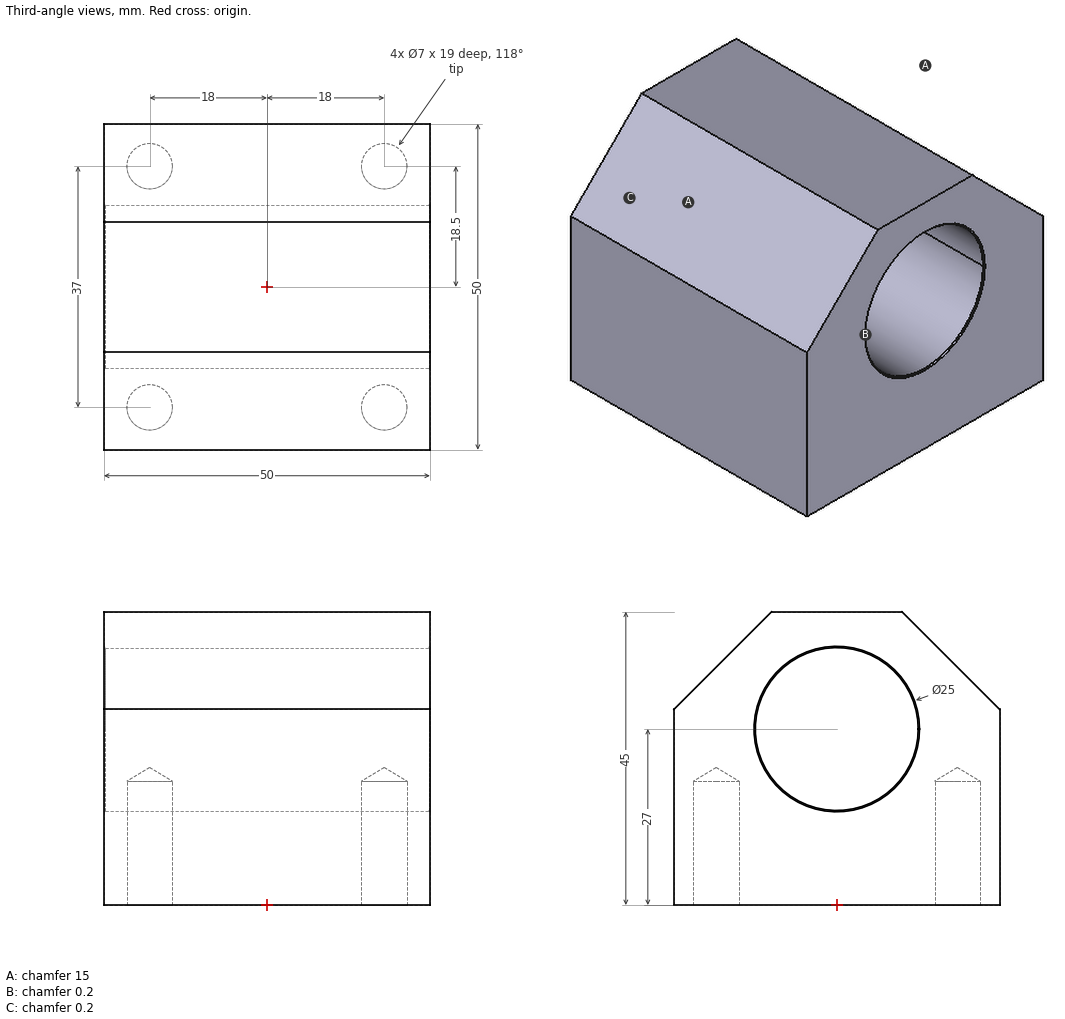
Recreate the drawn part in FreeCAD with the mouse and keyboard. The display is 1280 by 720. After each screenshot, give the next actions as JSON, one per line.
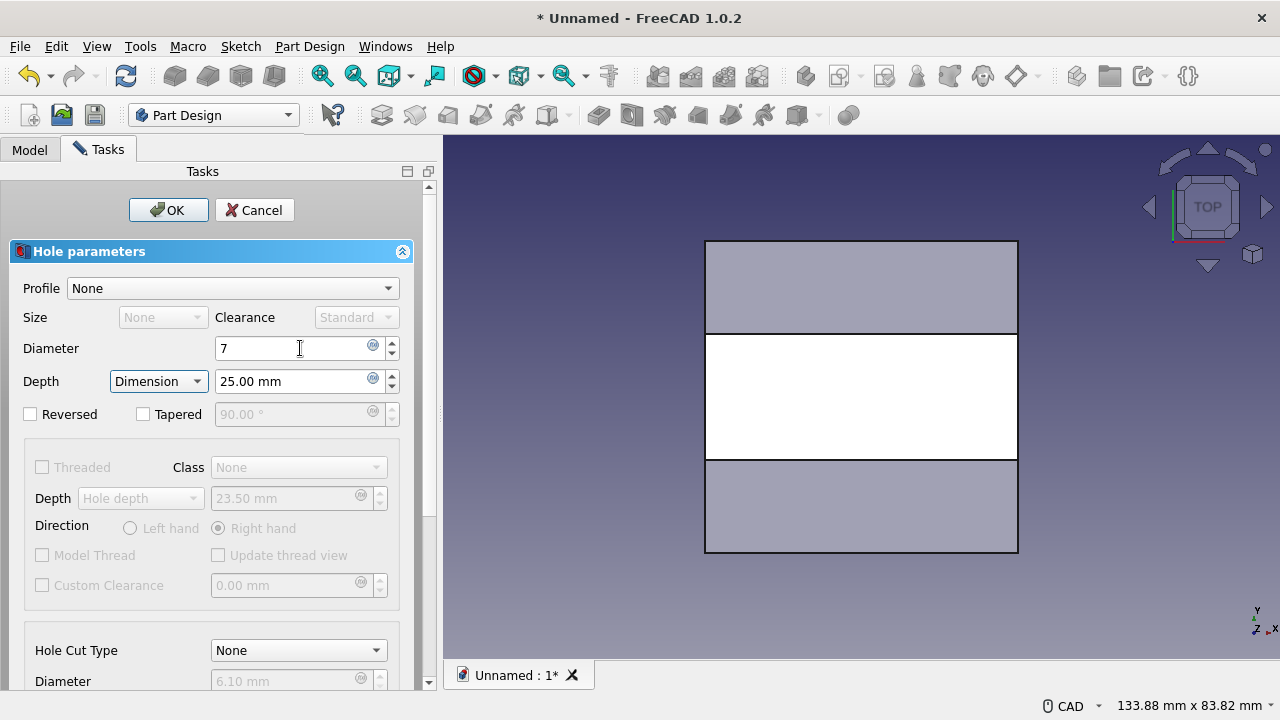
{"action": "triple_click", "coordinate": [300, 382]}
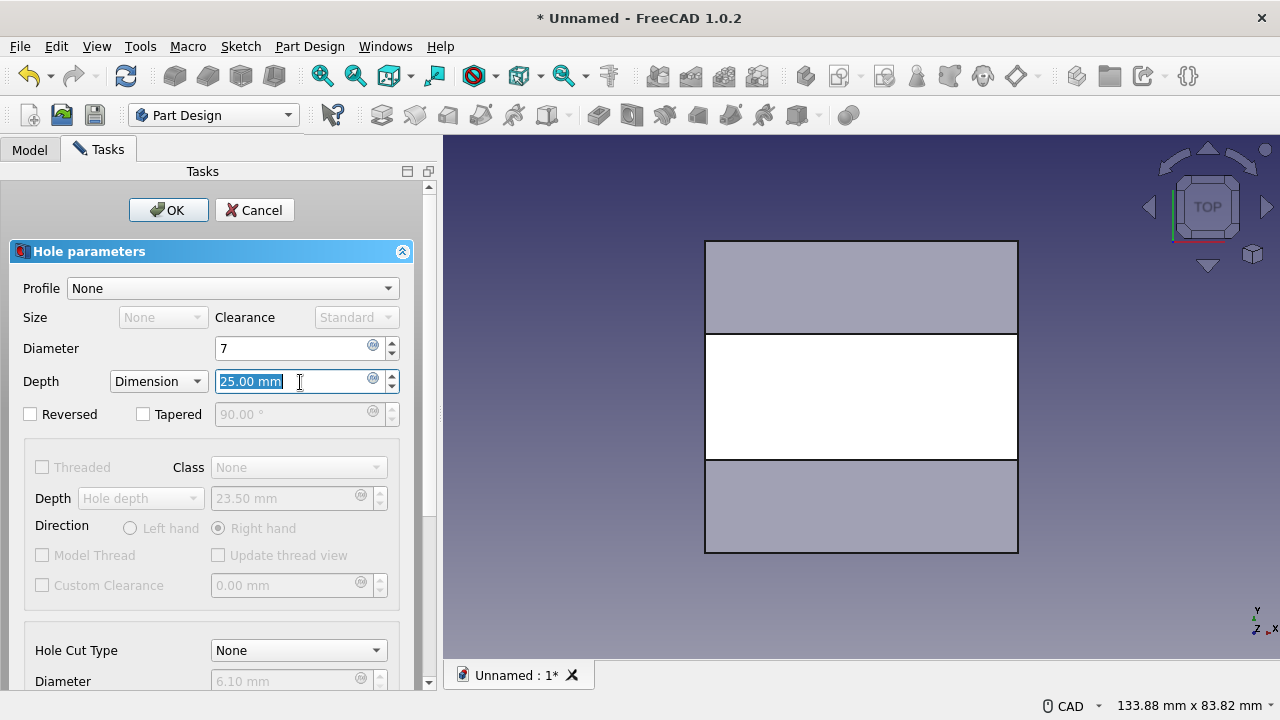
{"action": "type", "text": "19"}
{"action": "key", "text": "Tab"}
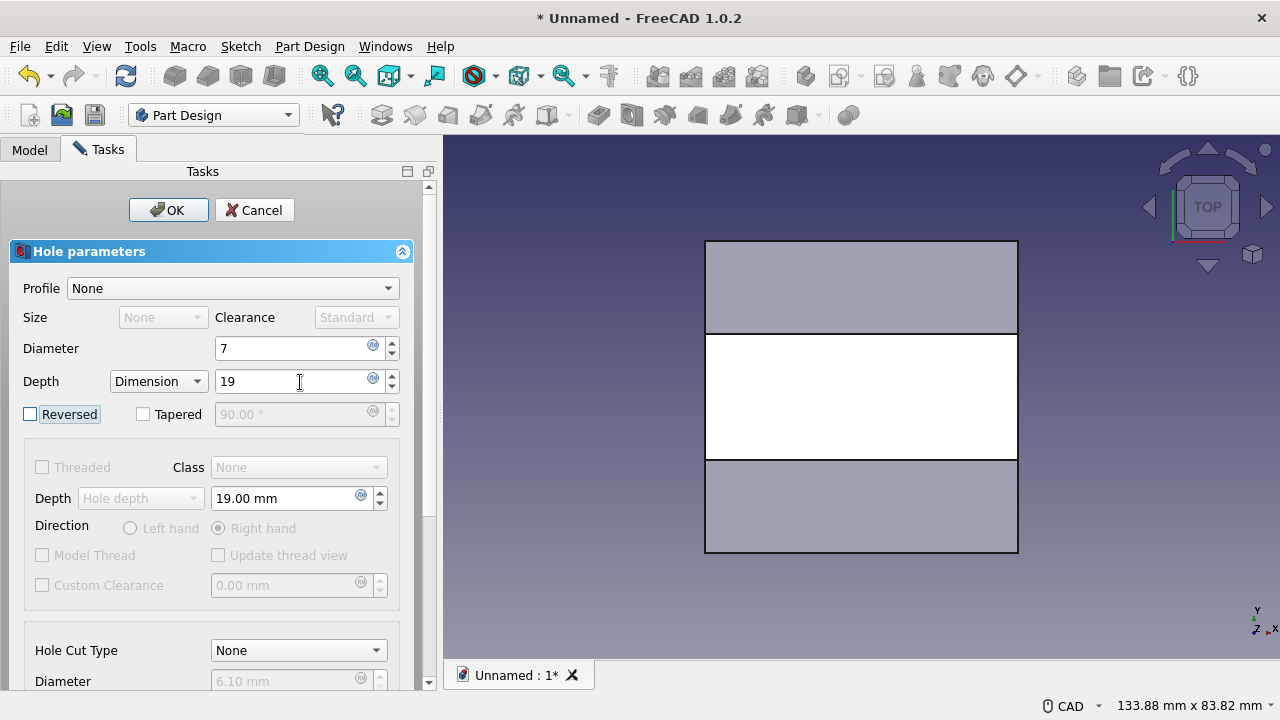
{"action": "left_click", "coordinate": [31, 414]}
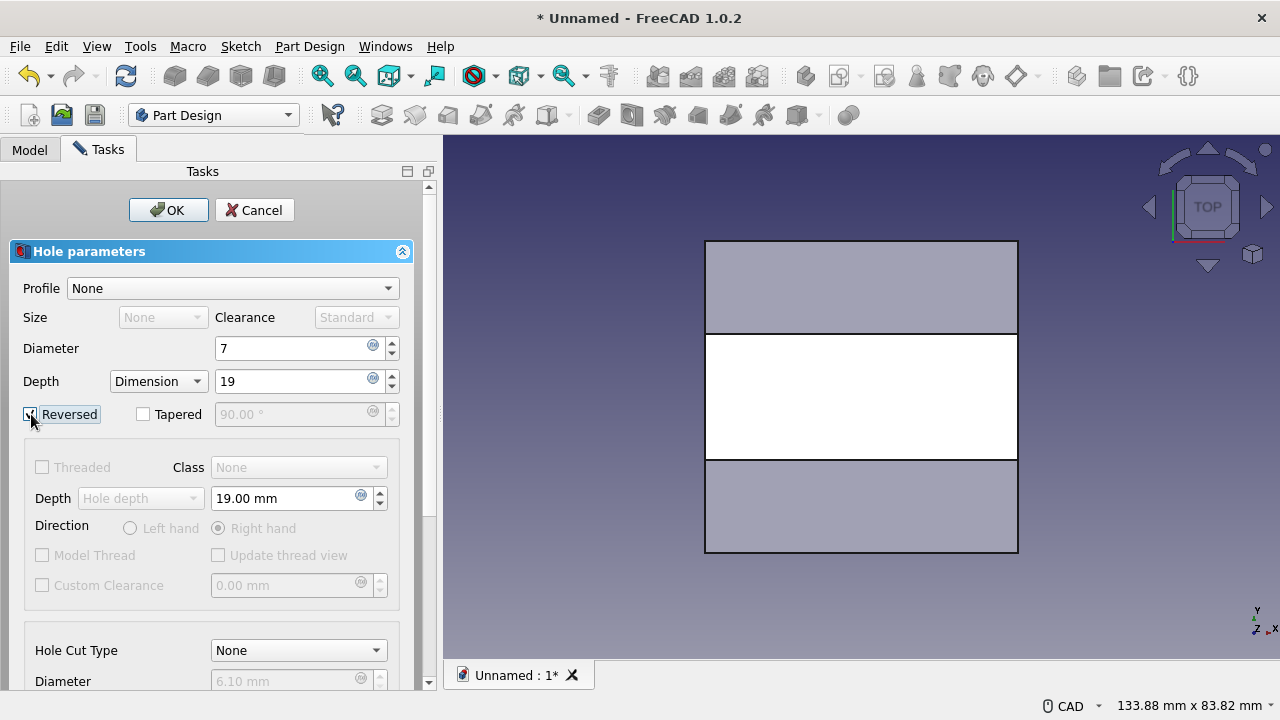
{"action": "left_click", "coordinate": [169, 210]}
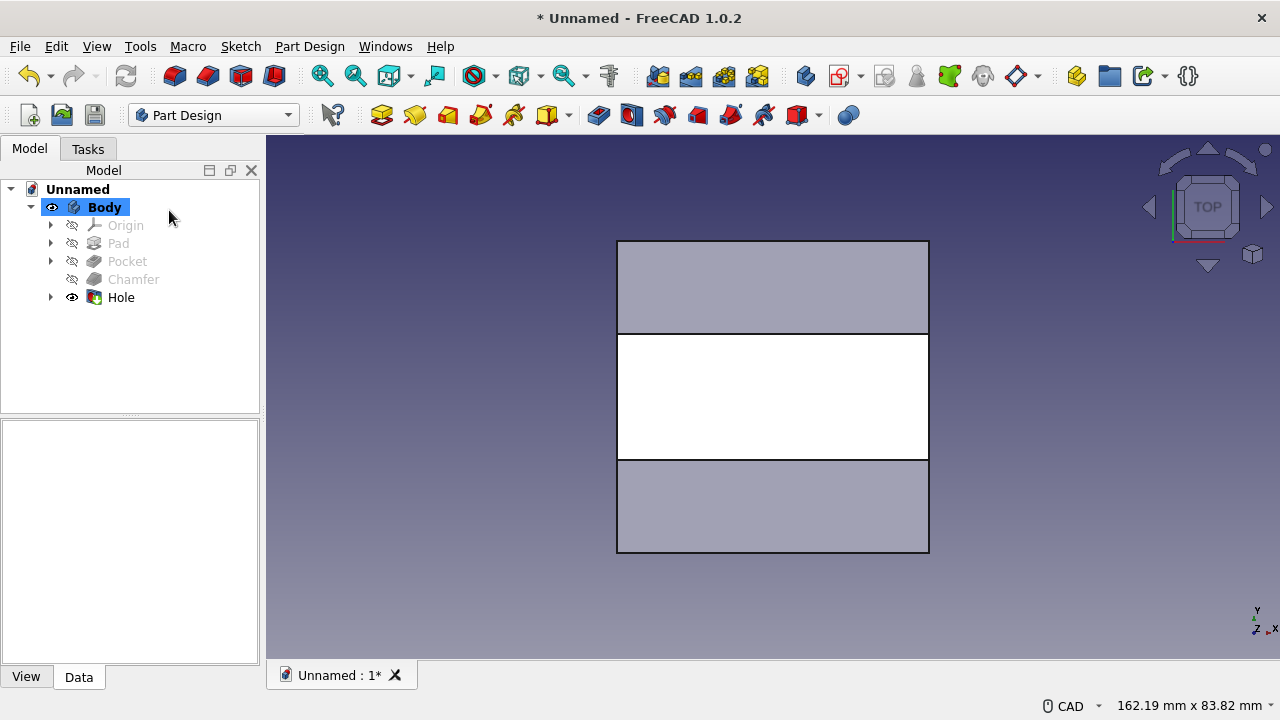
{"action": "key", "text": "0"}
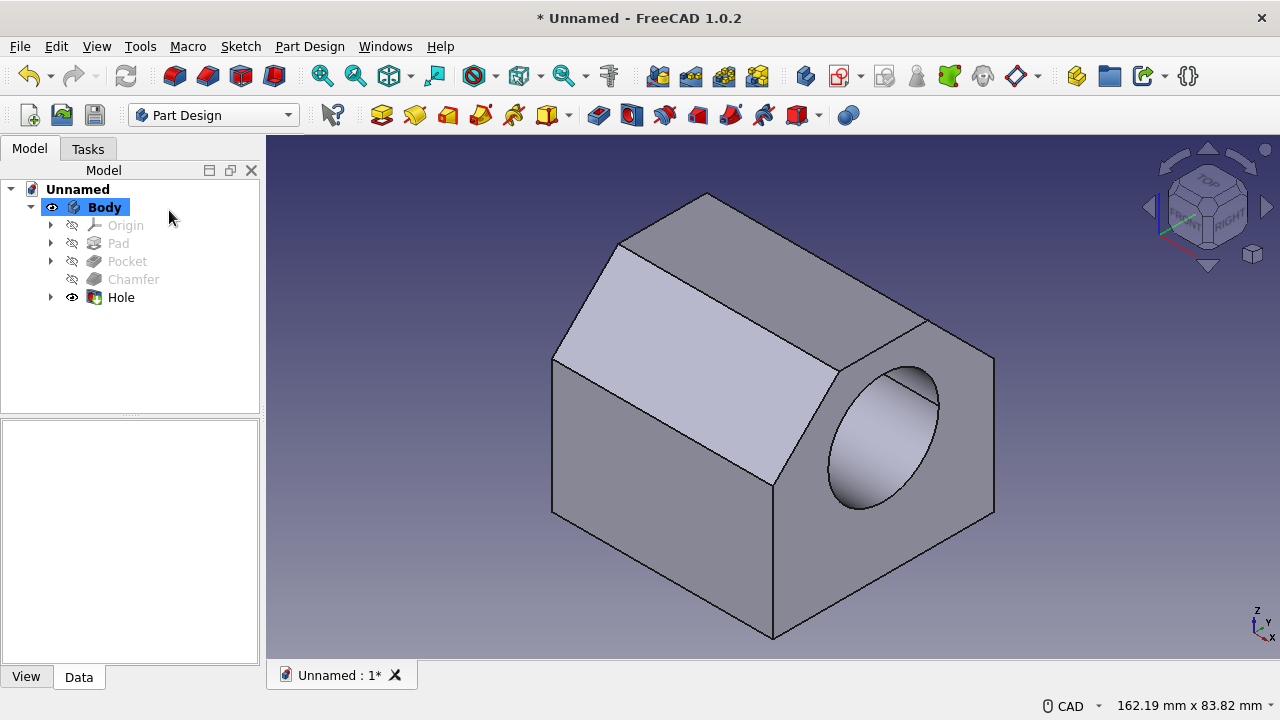
{"action": "left_click", "coordinate": [866, 507]}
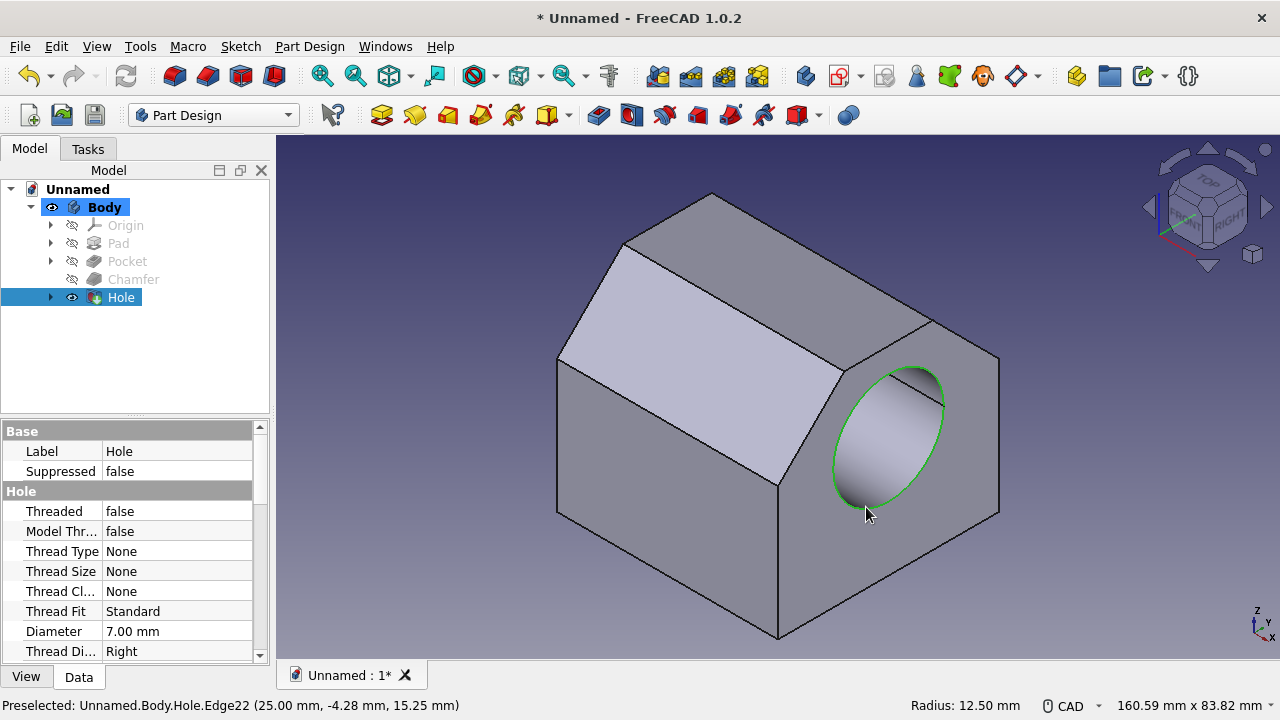
{"action": "left_click", "coordinate": [208, 76]}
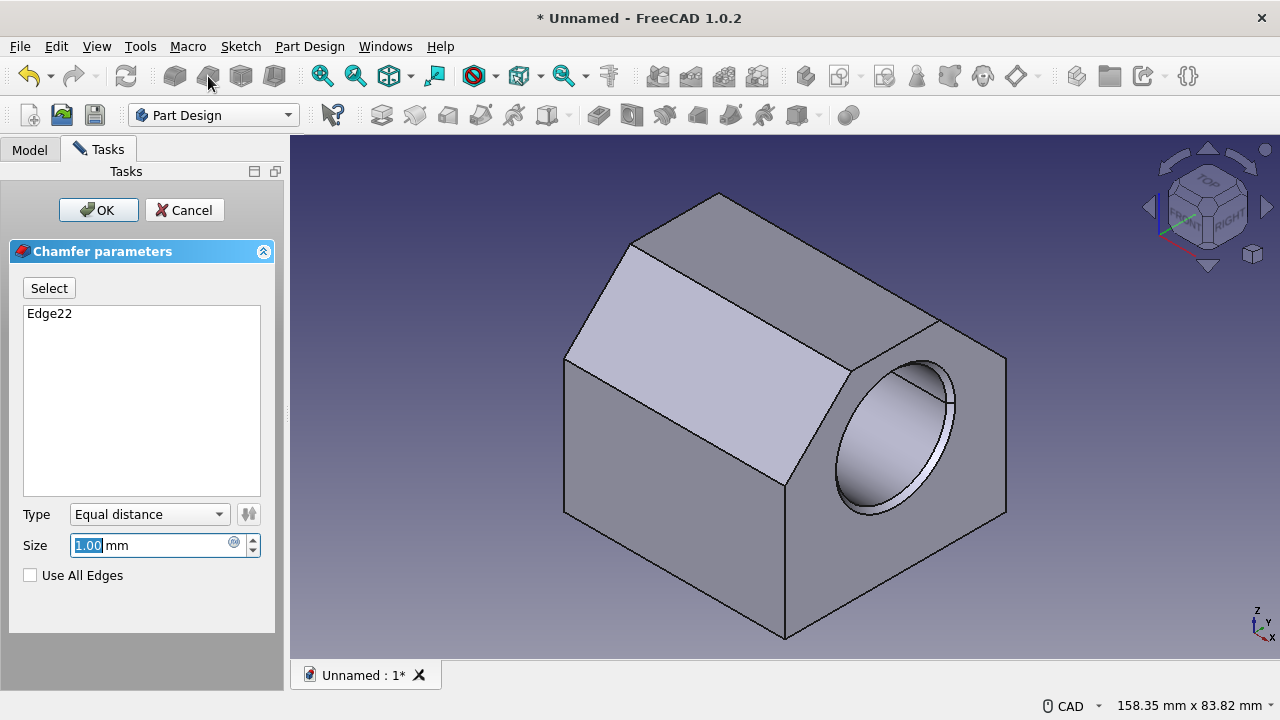
{"action": "type", "text": "0.2"}
{"action": "key", "text": "Tab"}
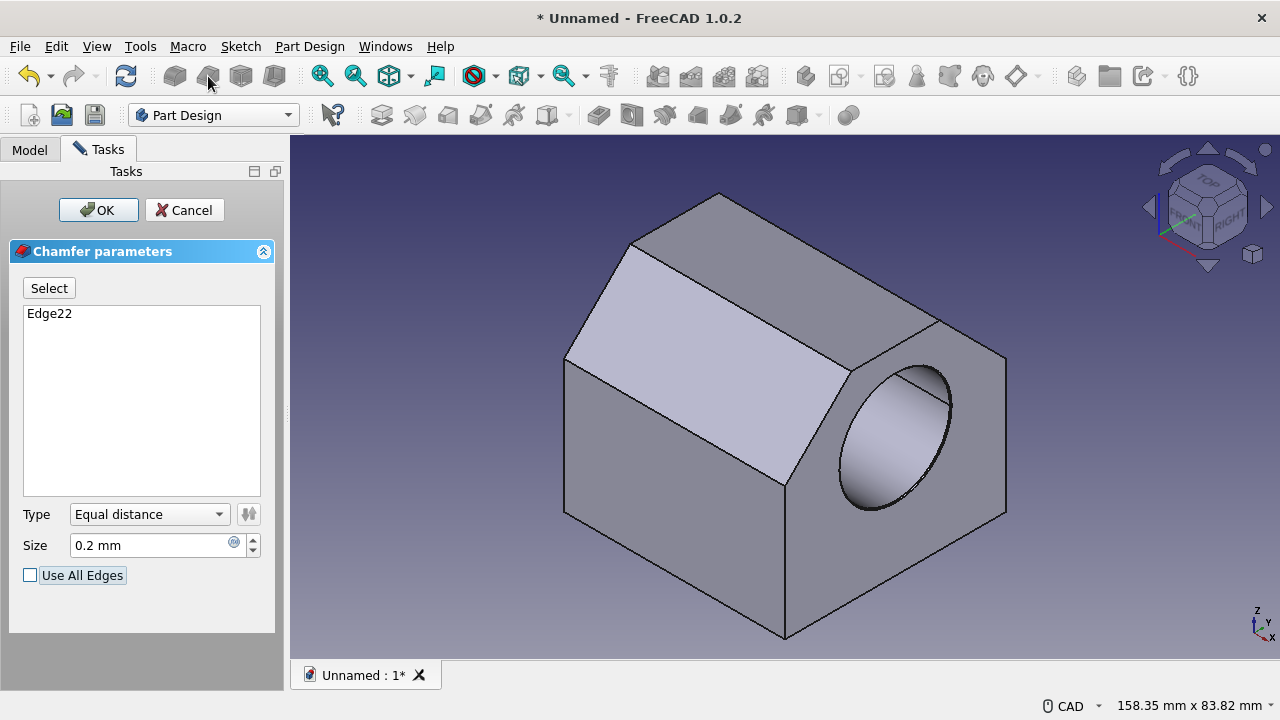
{"action": "left_click", "coordinate": [99, 210]}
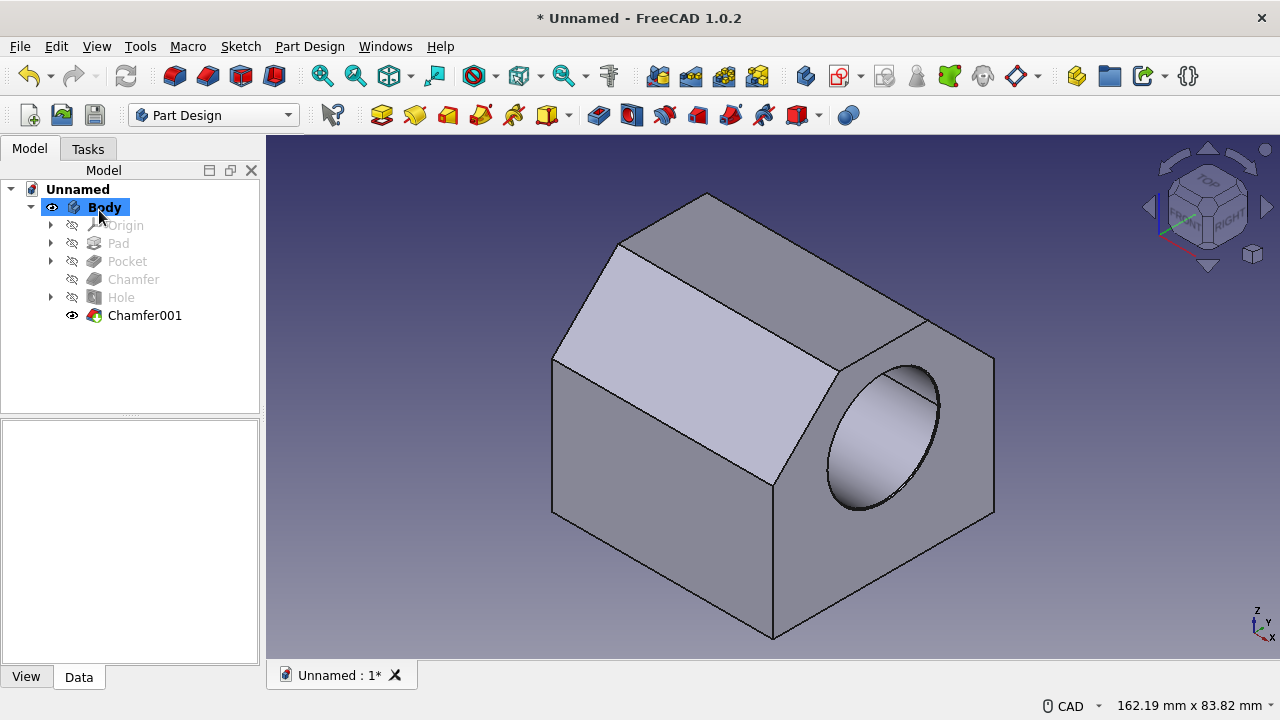
{"action": "key", "text": "2"}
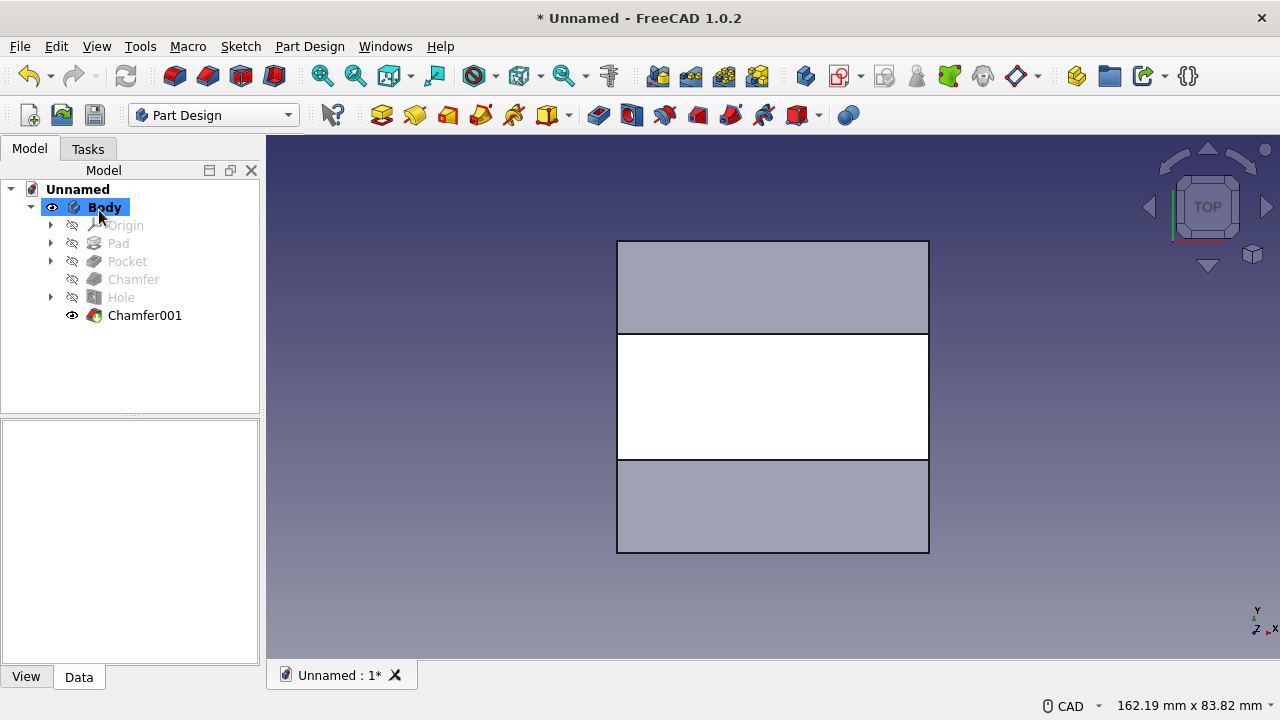
{"action": "key", "text": "0"}